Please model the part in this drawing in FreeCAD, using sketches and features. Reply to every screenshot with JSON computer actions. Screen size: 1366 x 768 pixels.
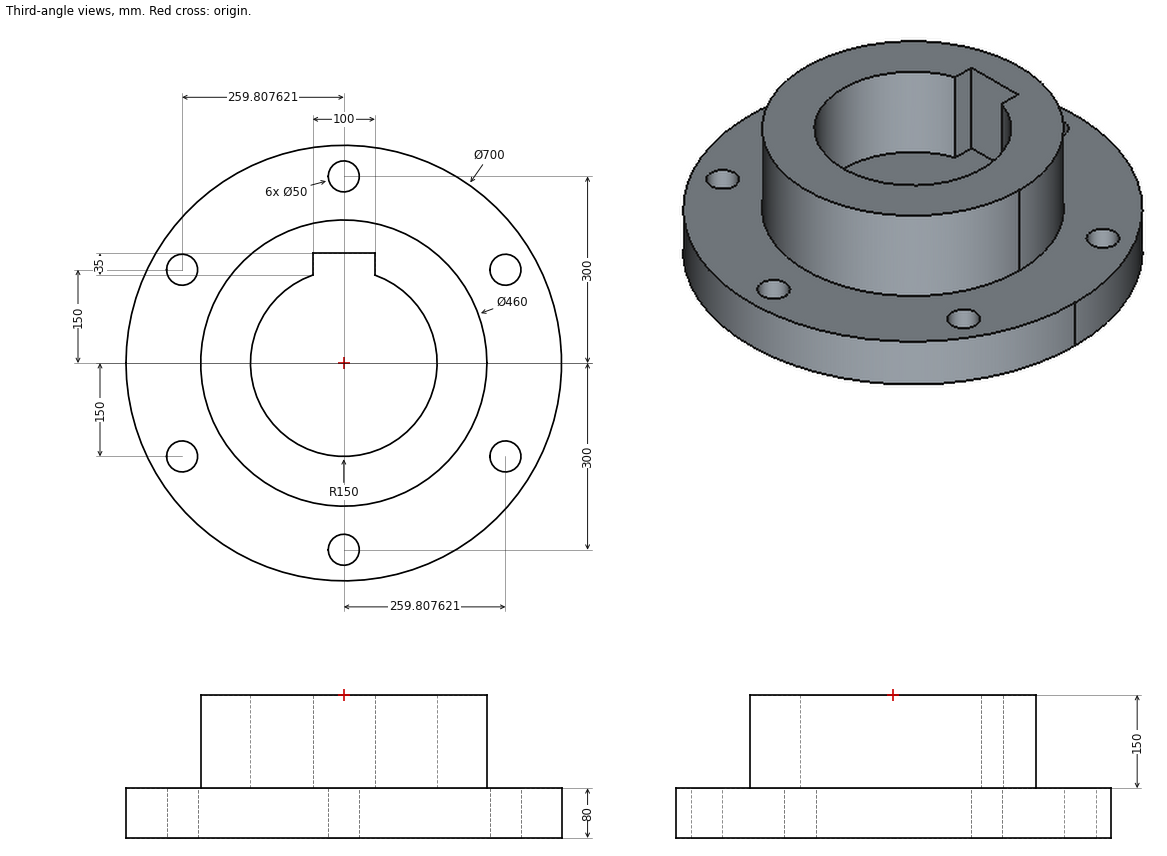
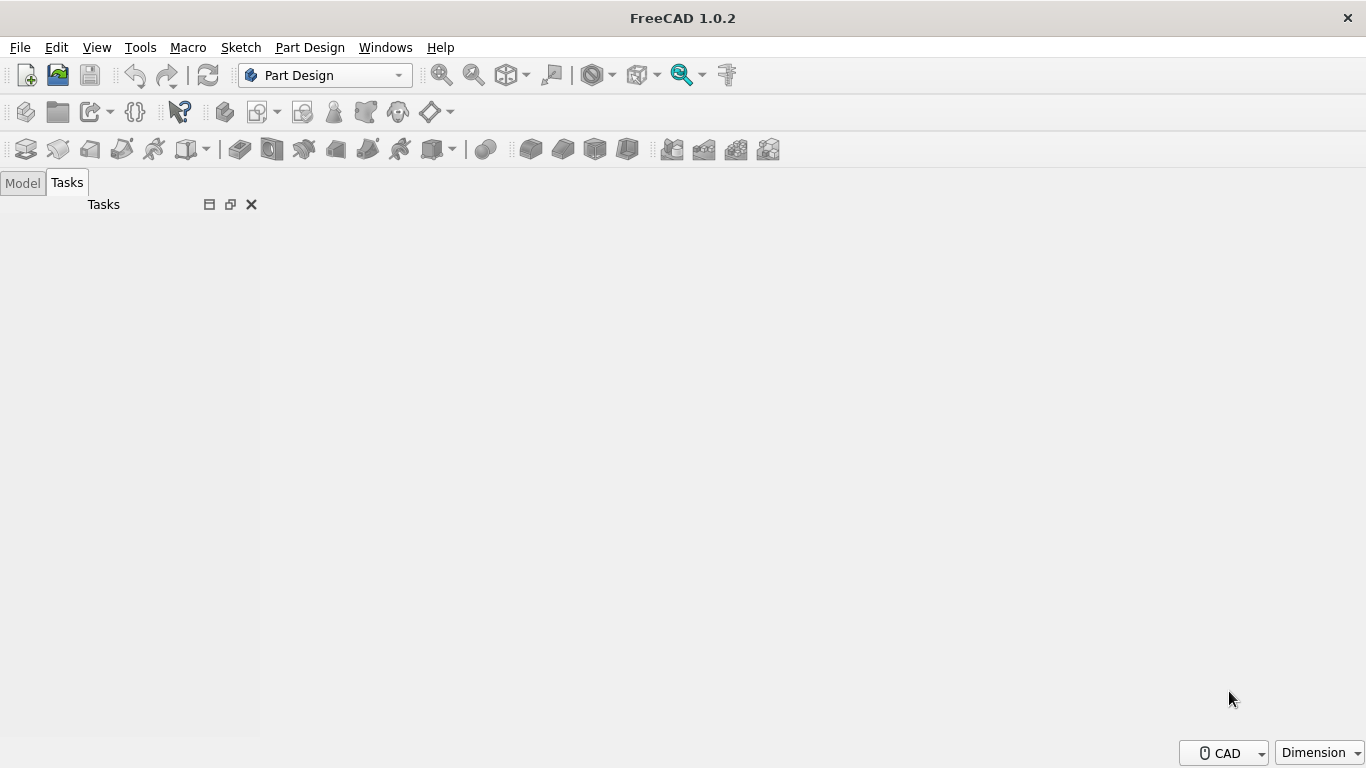
{"action": "key", "text": "ctrl+n"}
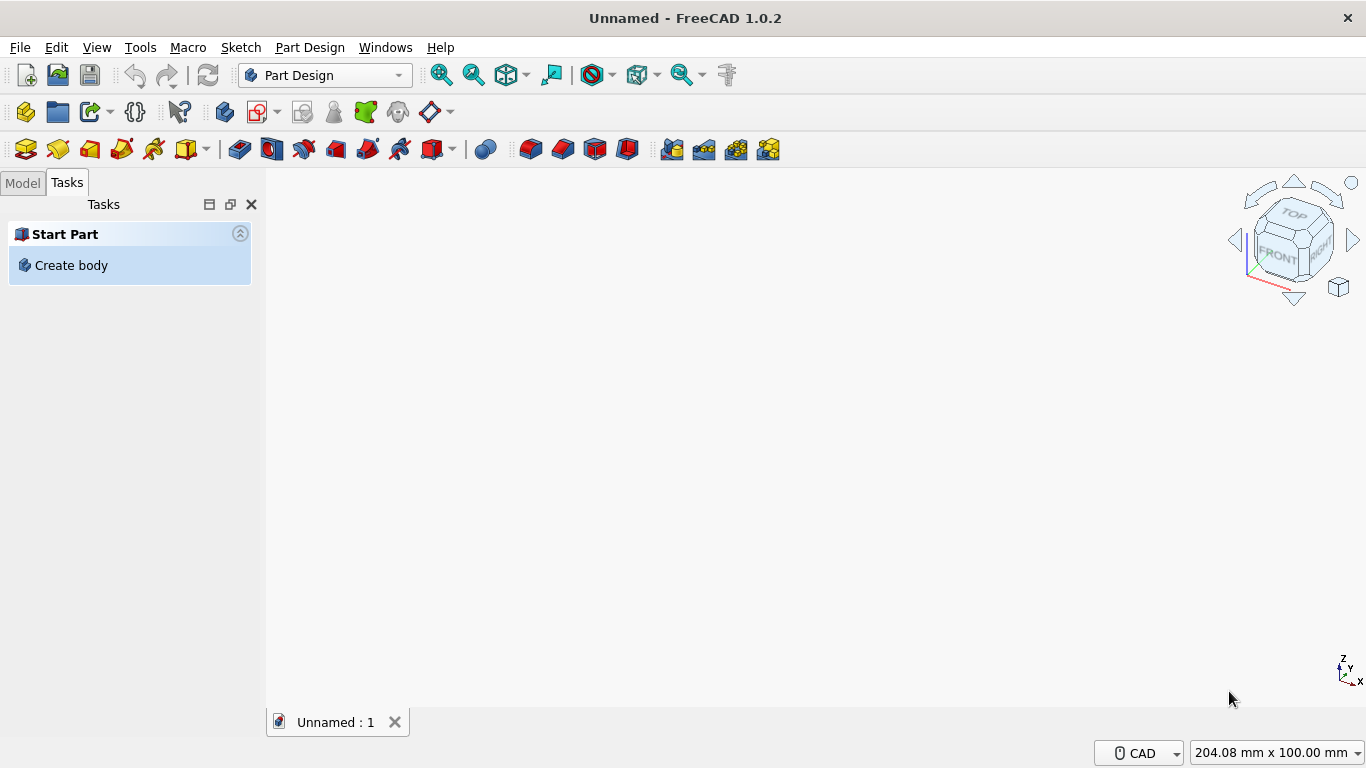
{"action": "left_click", "coordinate": [258, 112]}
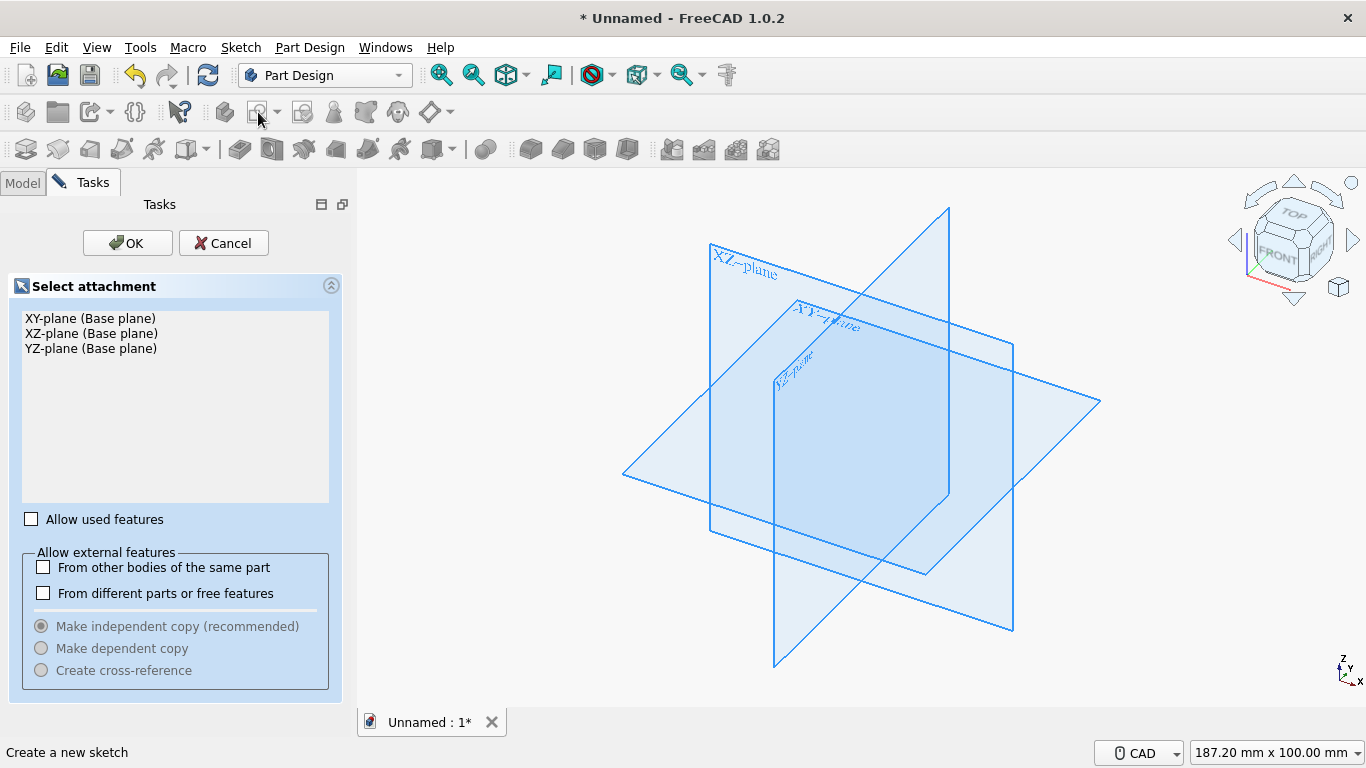
{"action": "left_click", "coordinate": [82, 318]}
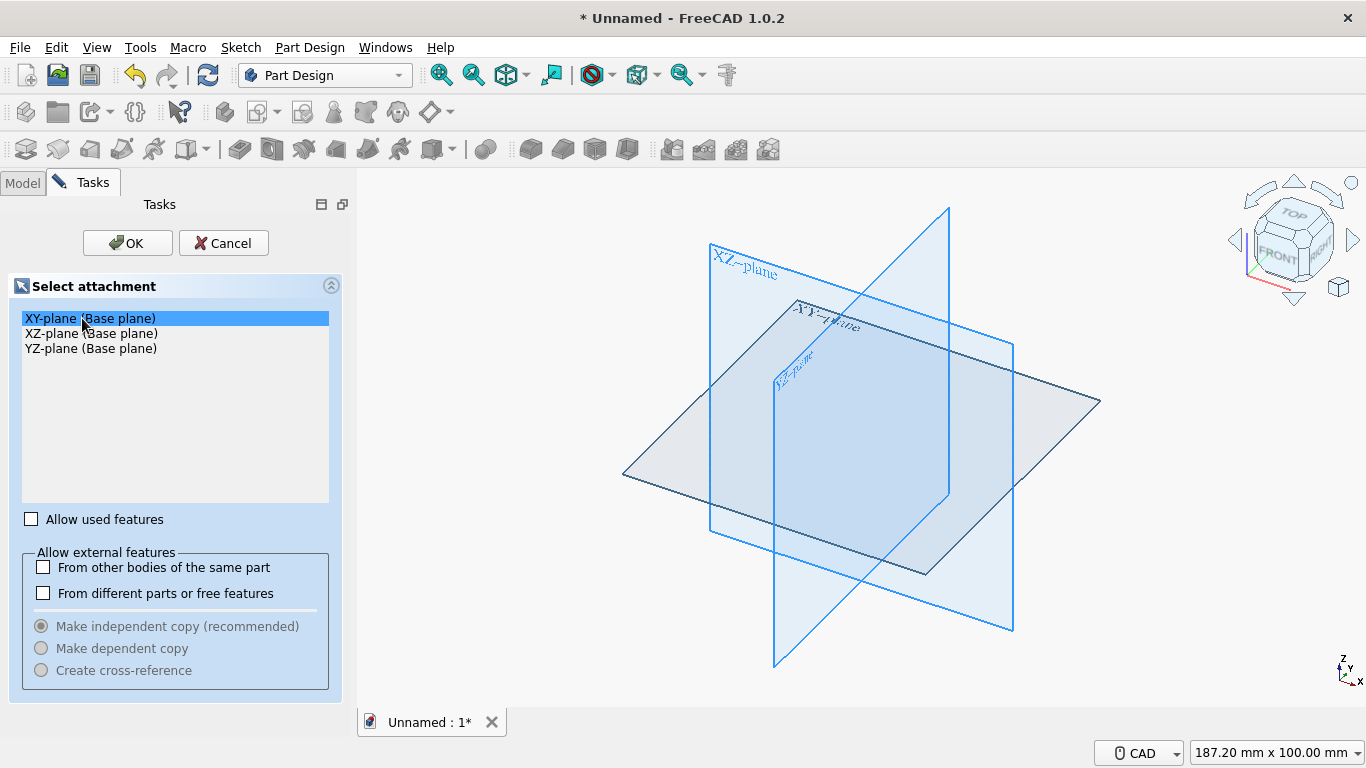
{"action": "left_click", "coordinate": [128, 243]}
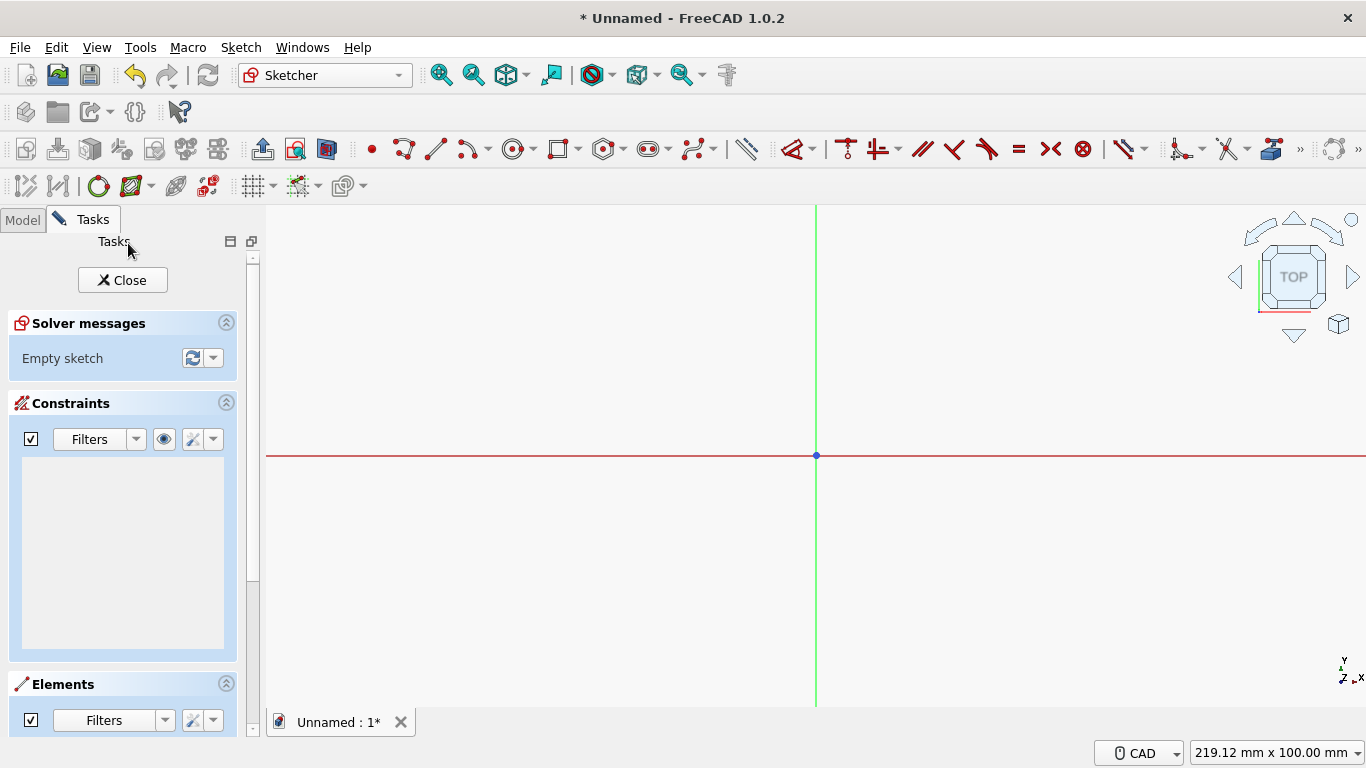
{"action": "scroll", "coordinate": [737, 456], "scroll_direction": "down", "scroll_amount": 10}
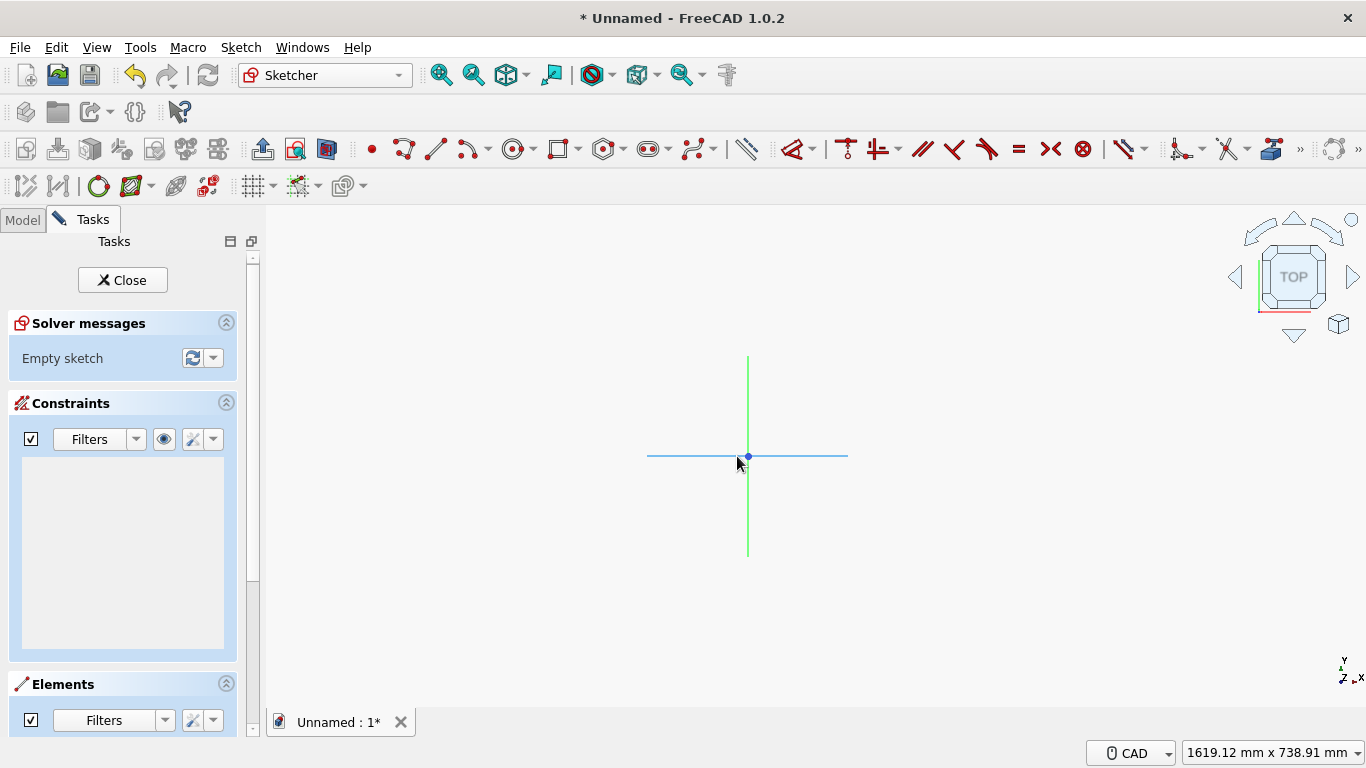
{"action": "key", "text": "g m"}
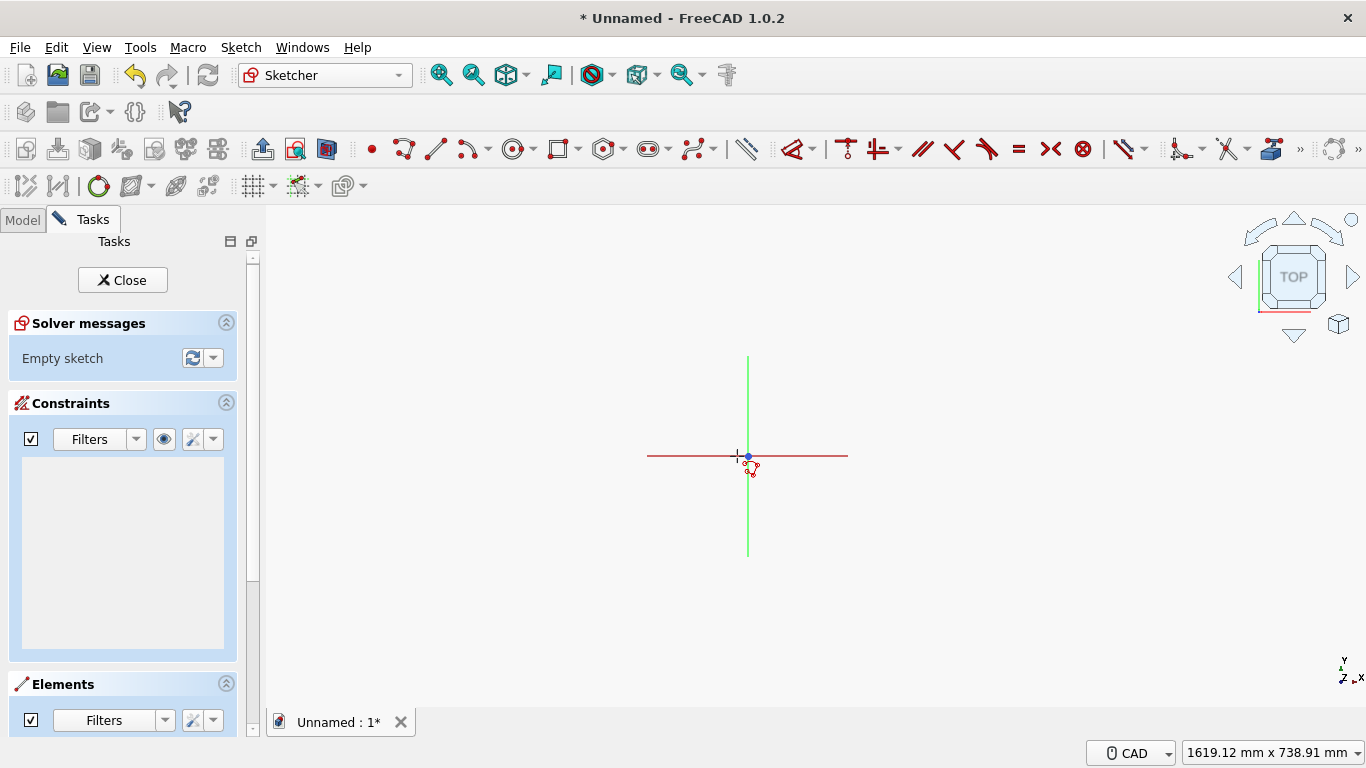
{"action": "left_click", "coordinate": [714, 360]}
{"action": "left_click", "coordinate": [714, 337]}
{"action": "left_click", "coordinate": [782, 337]}
{"action": "left_click", "coordinate": [782, 360]}
{"action": "right_click", "coordinate": [782, 360]}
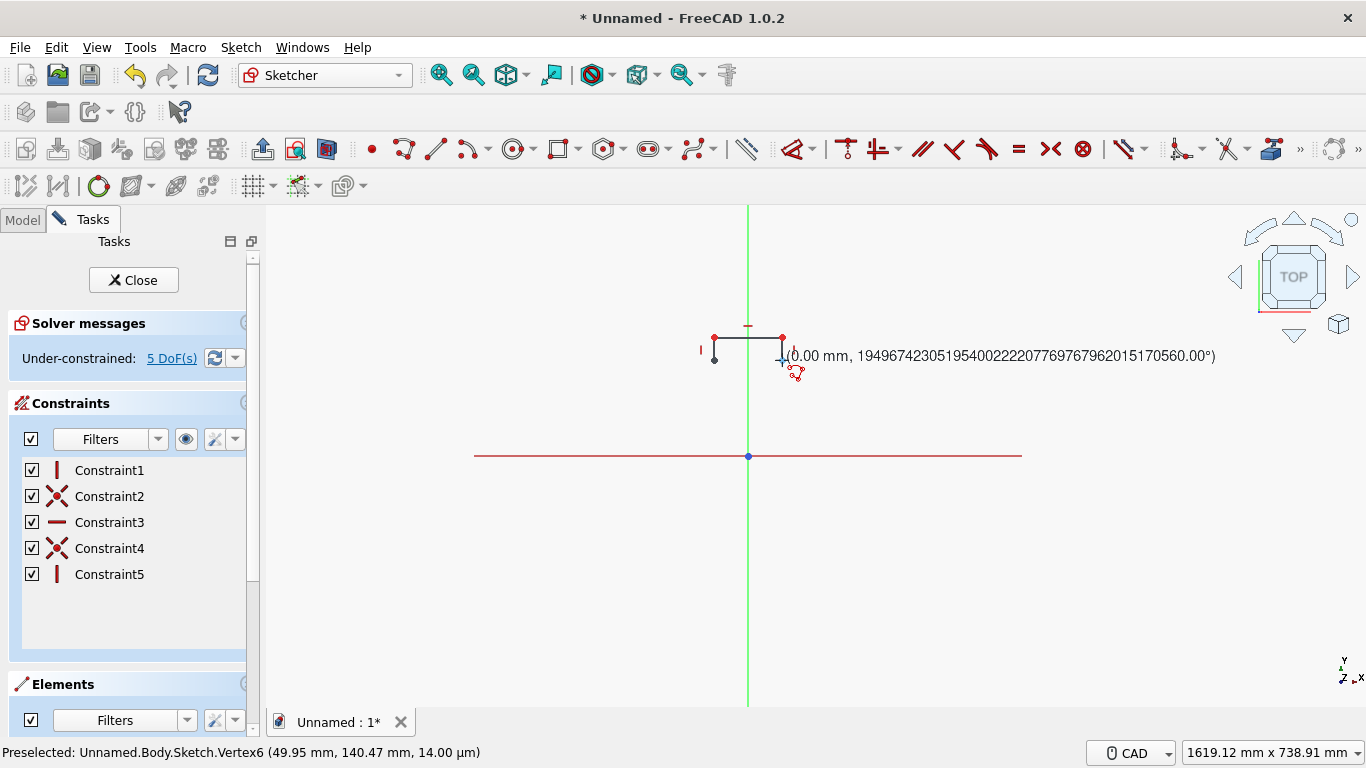
{"action": "left_click", "coordinate": [490, 150]}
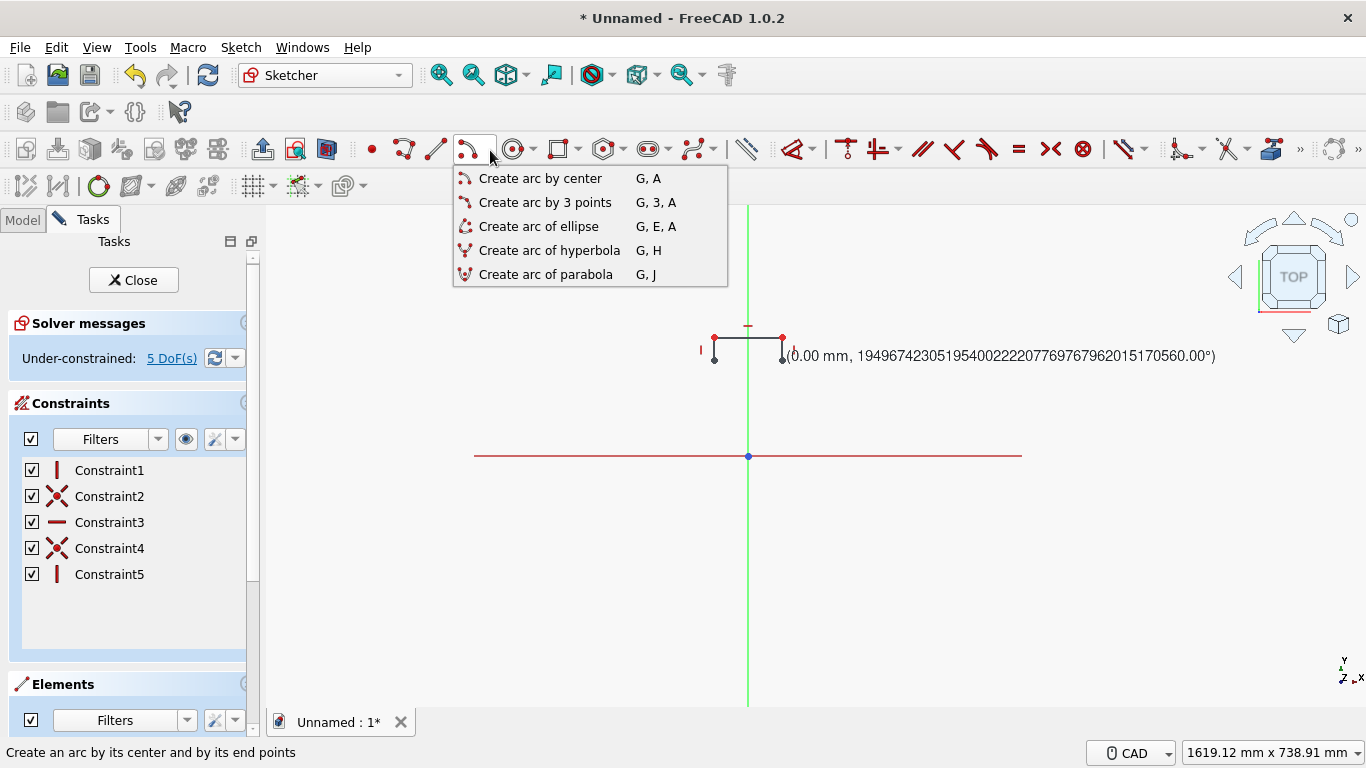
{"action": "left_click", "coordinate": [590, 202]}